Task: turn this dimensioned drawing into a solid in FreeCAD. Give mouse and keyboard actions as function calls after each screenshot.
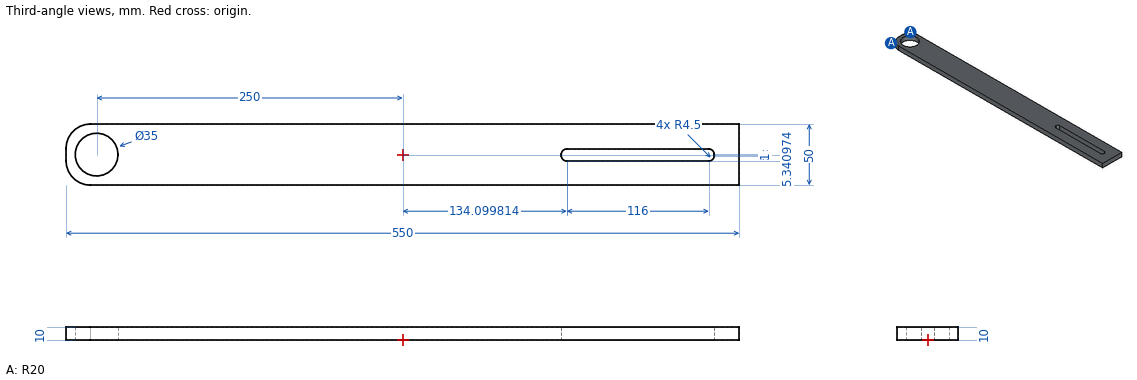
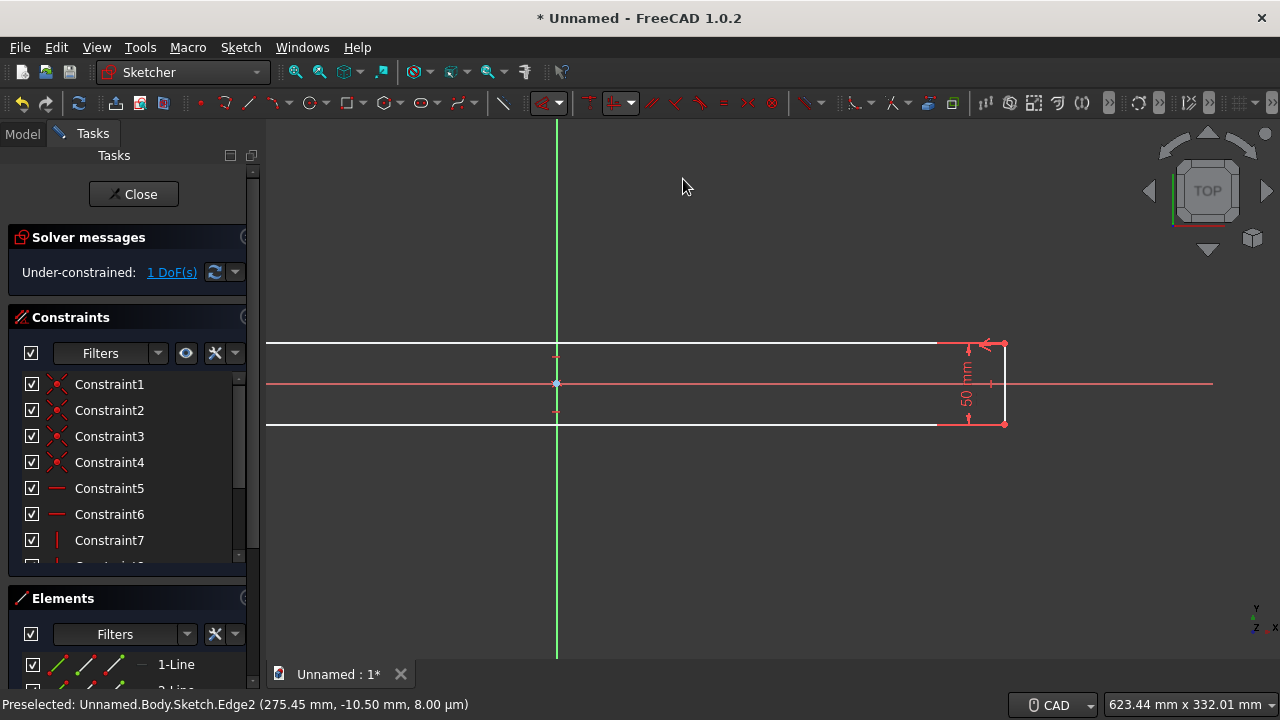
click(377, 425)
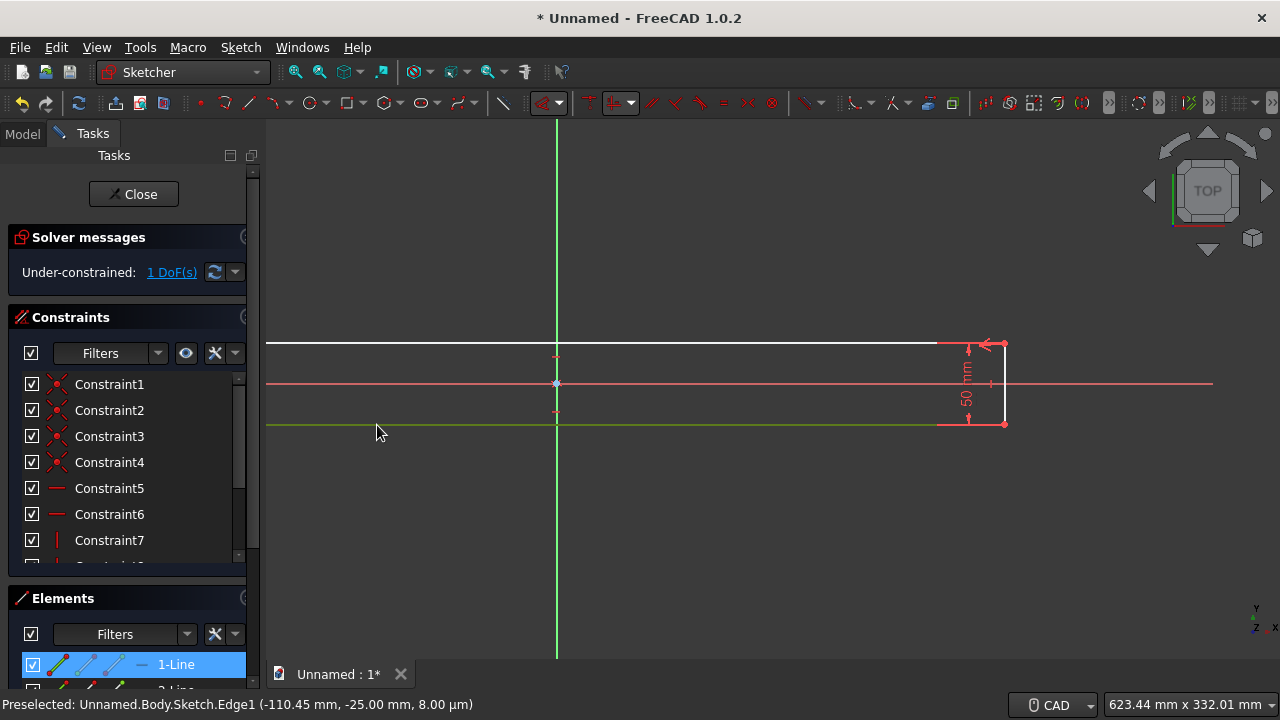
key(l)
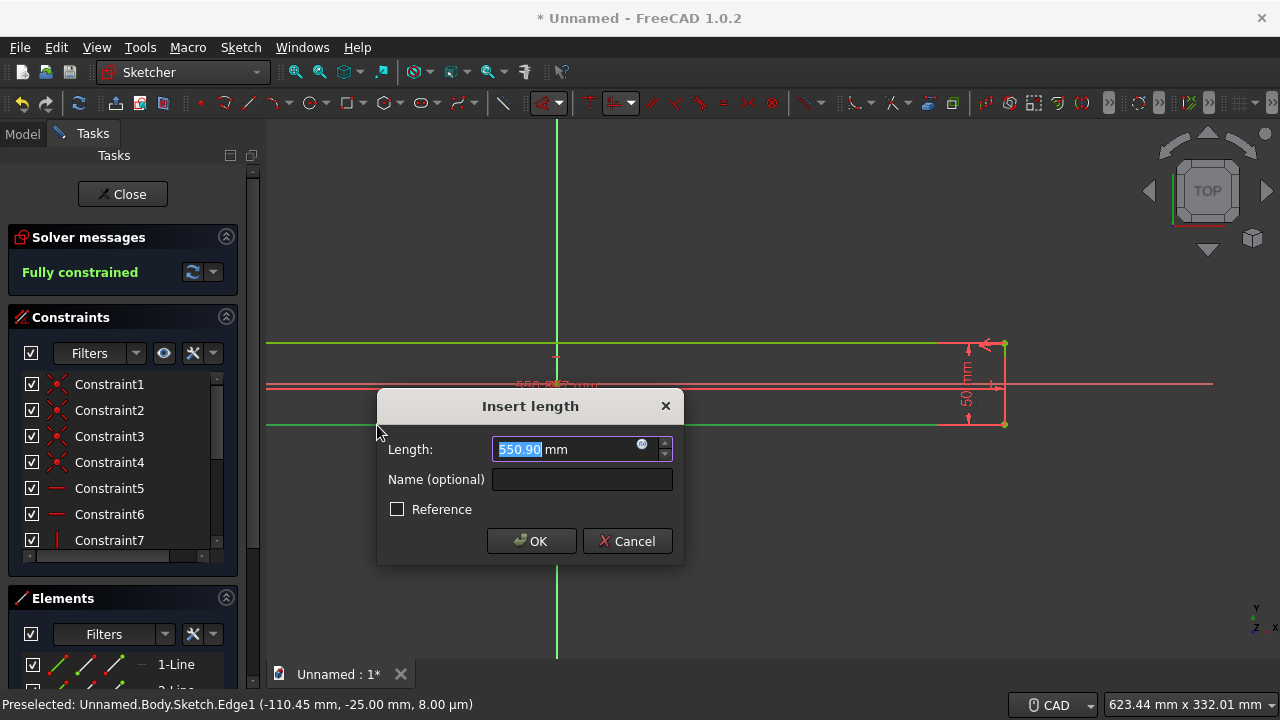
text(550)
key(Return)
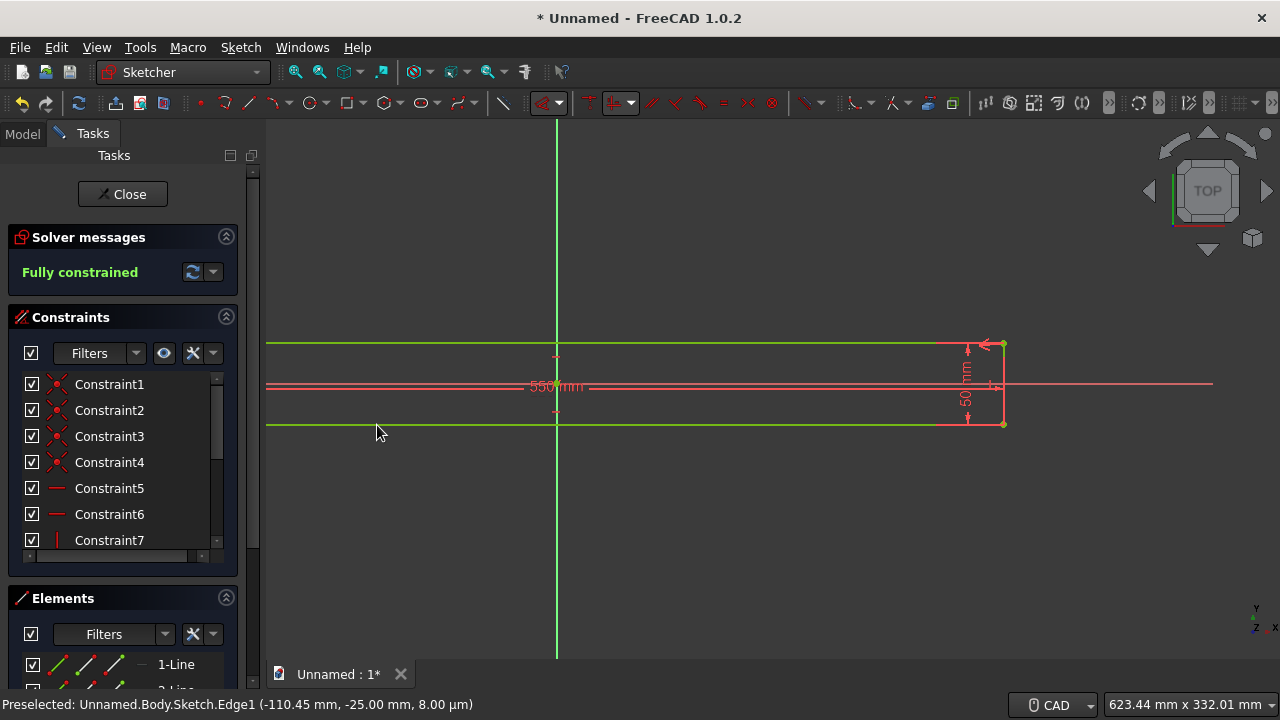
click(123, 194)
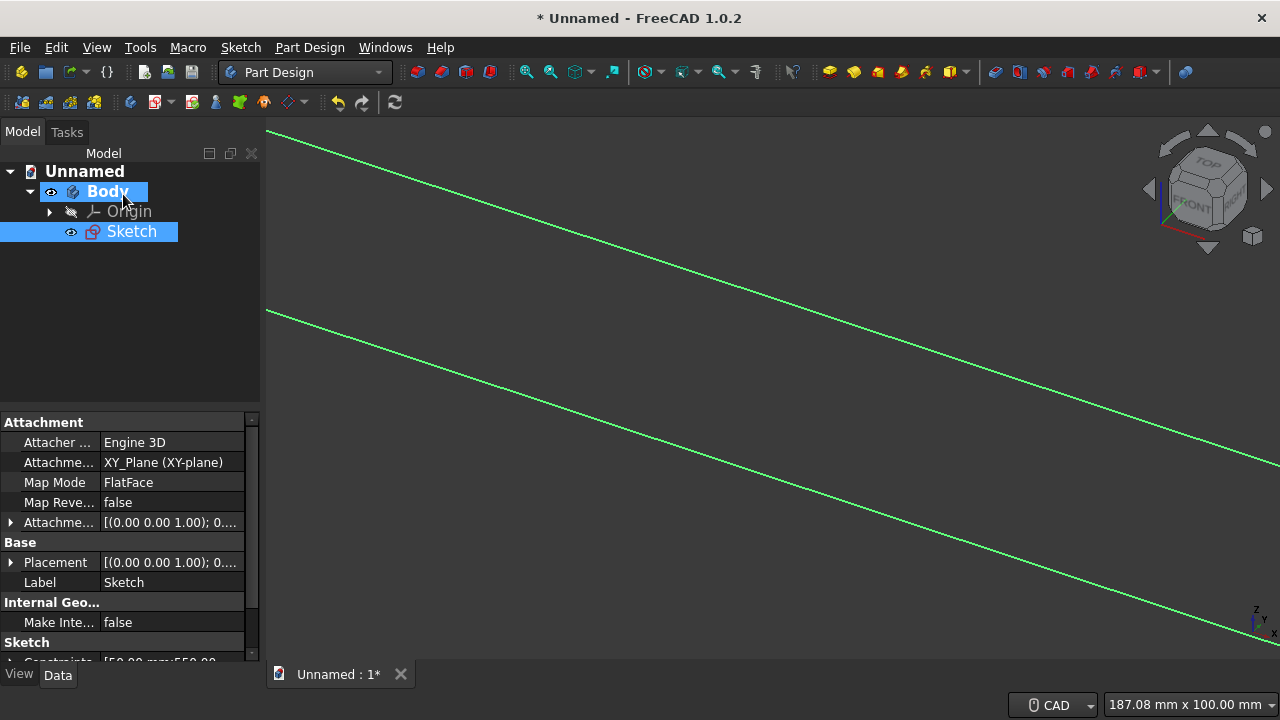
click(830, 72)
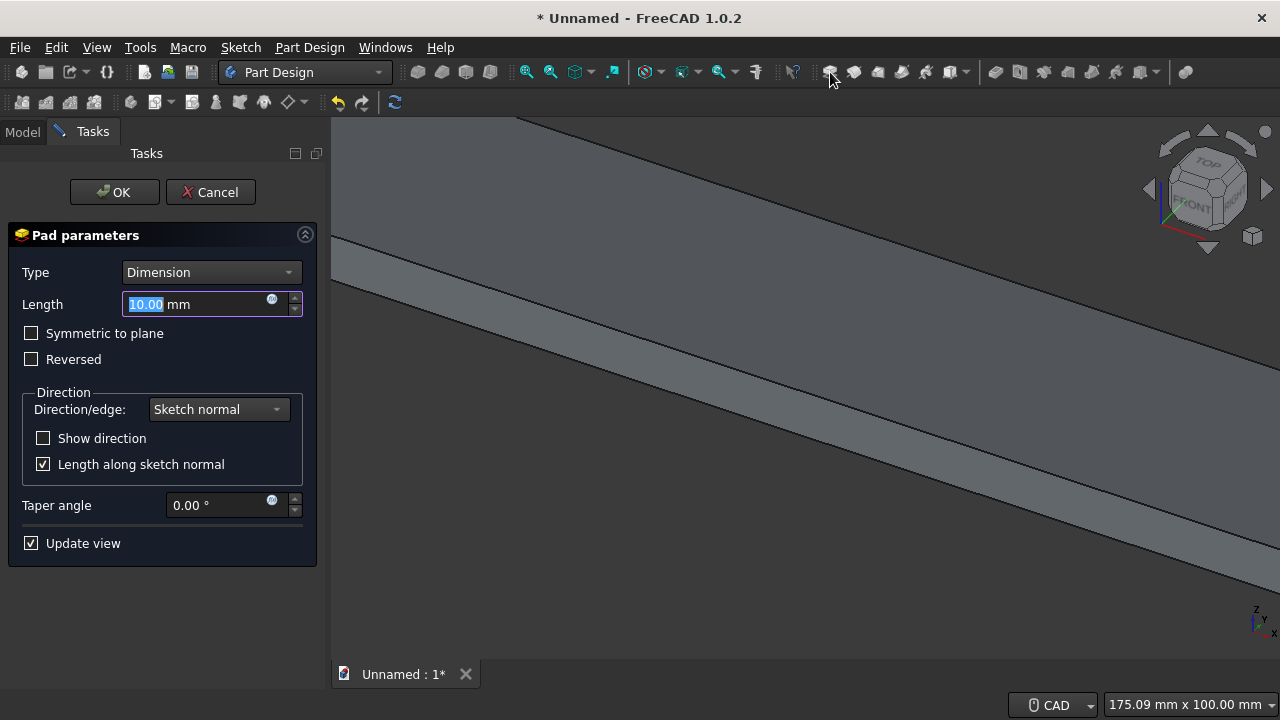
text(10)
key(Tab)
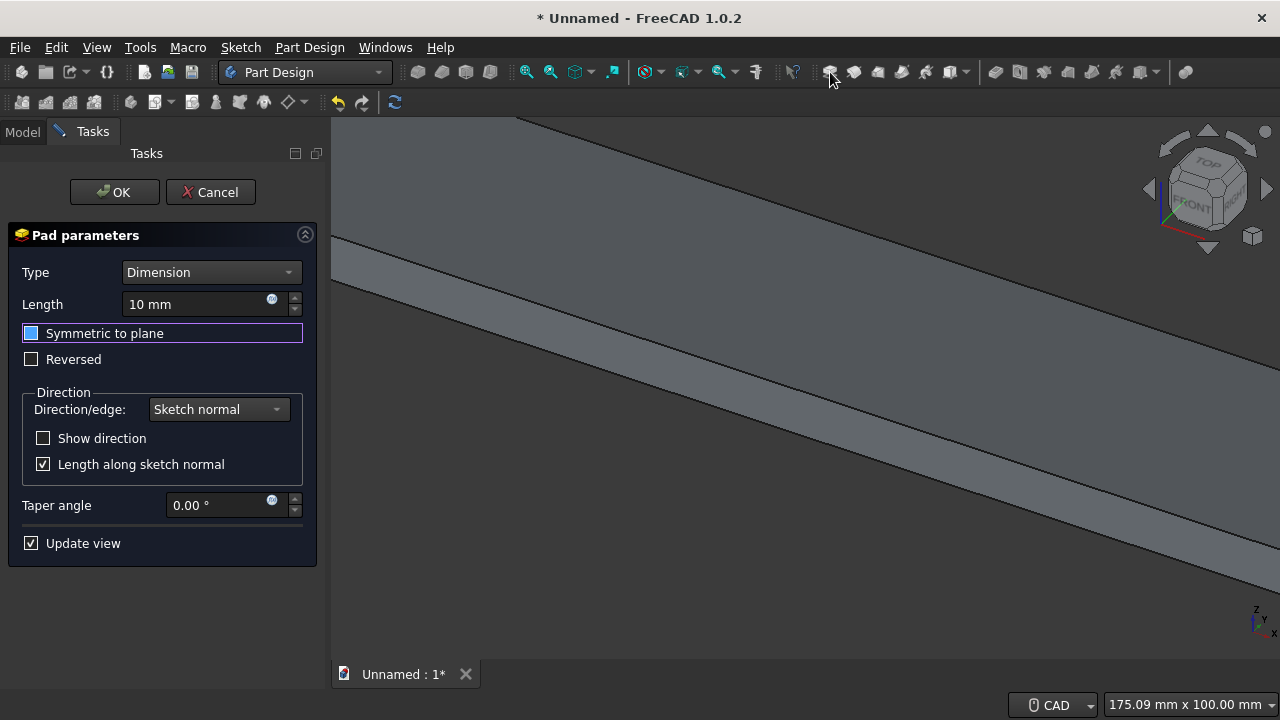
click(115, 192)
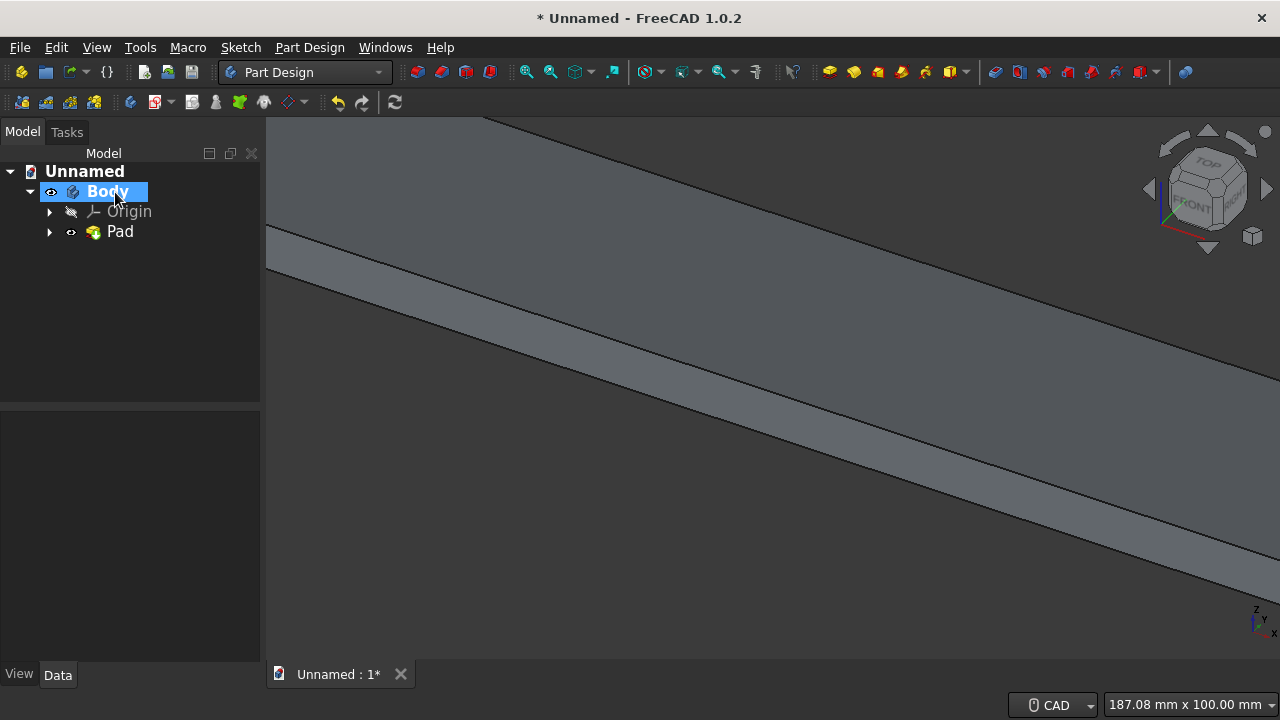
click(528, 72)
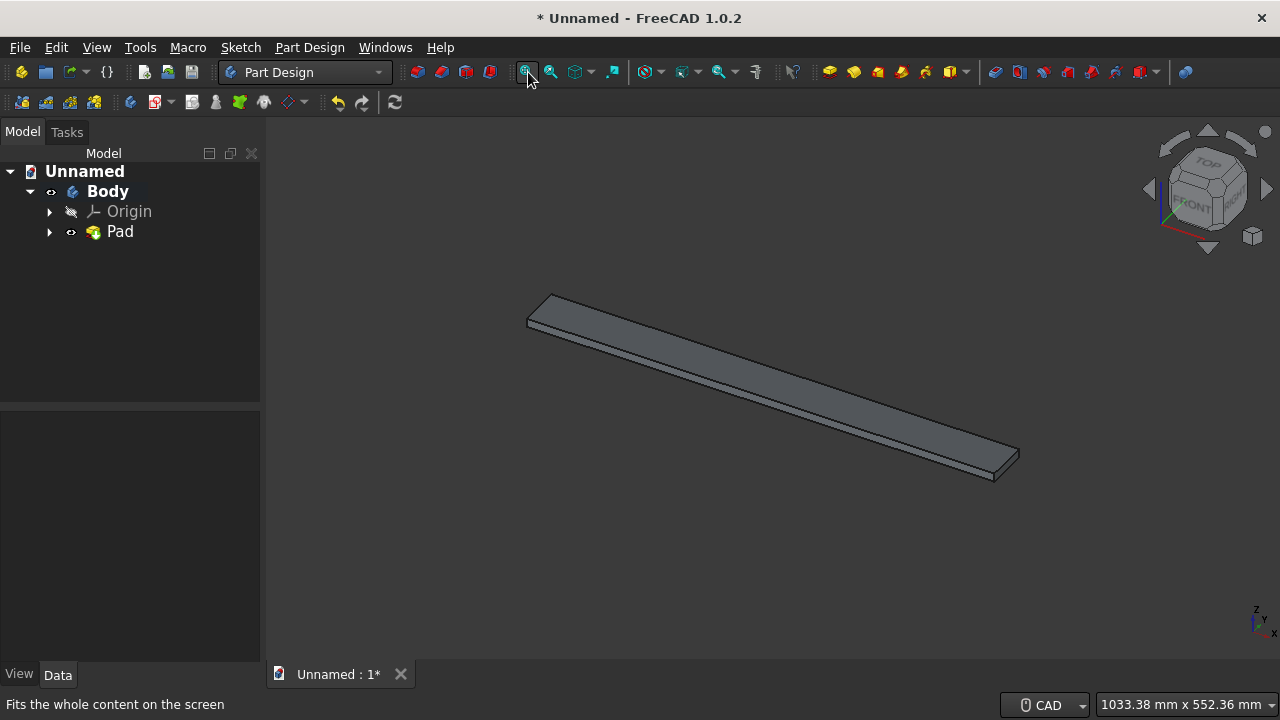
click(973, 449)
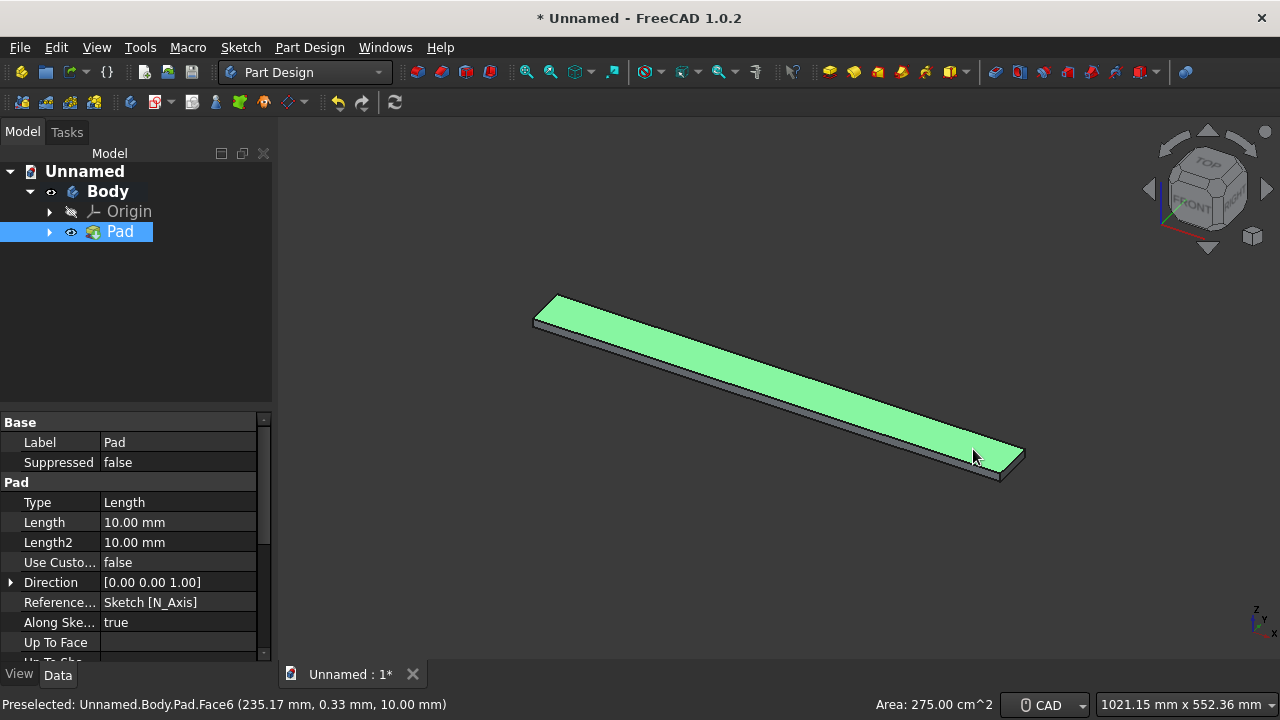
click(156, 102)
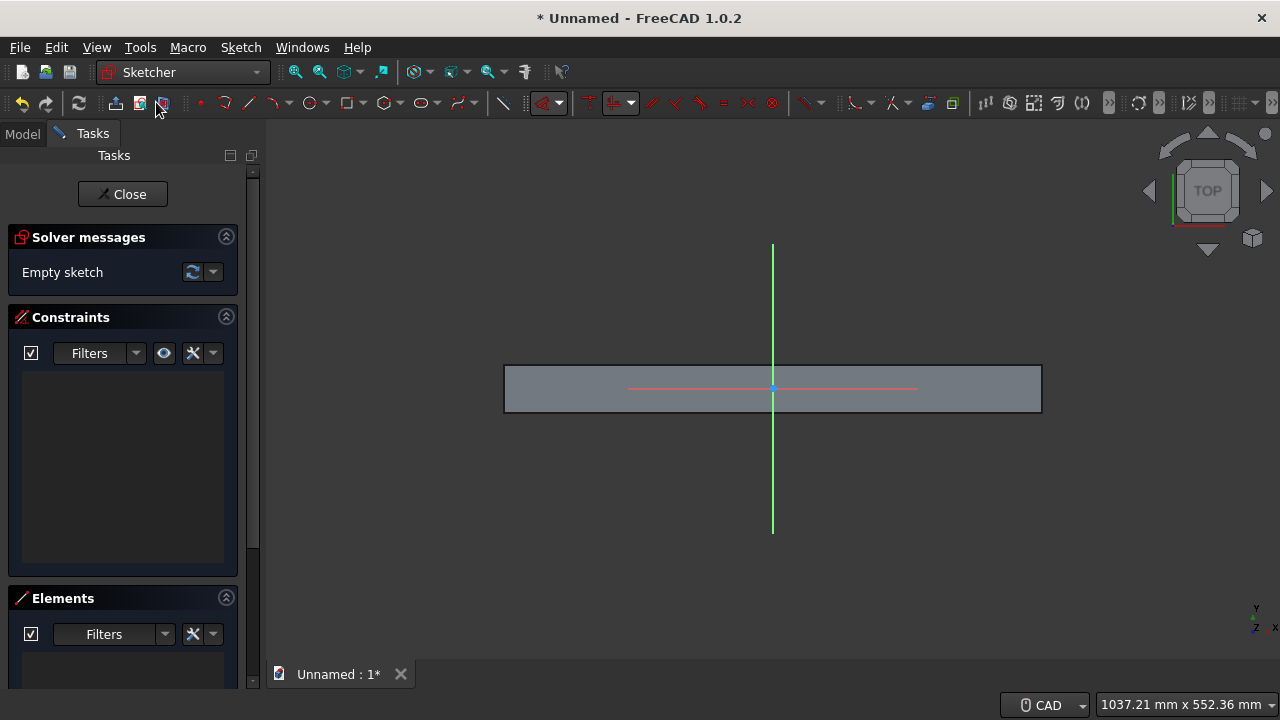
scroll(511, 389, up, 12)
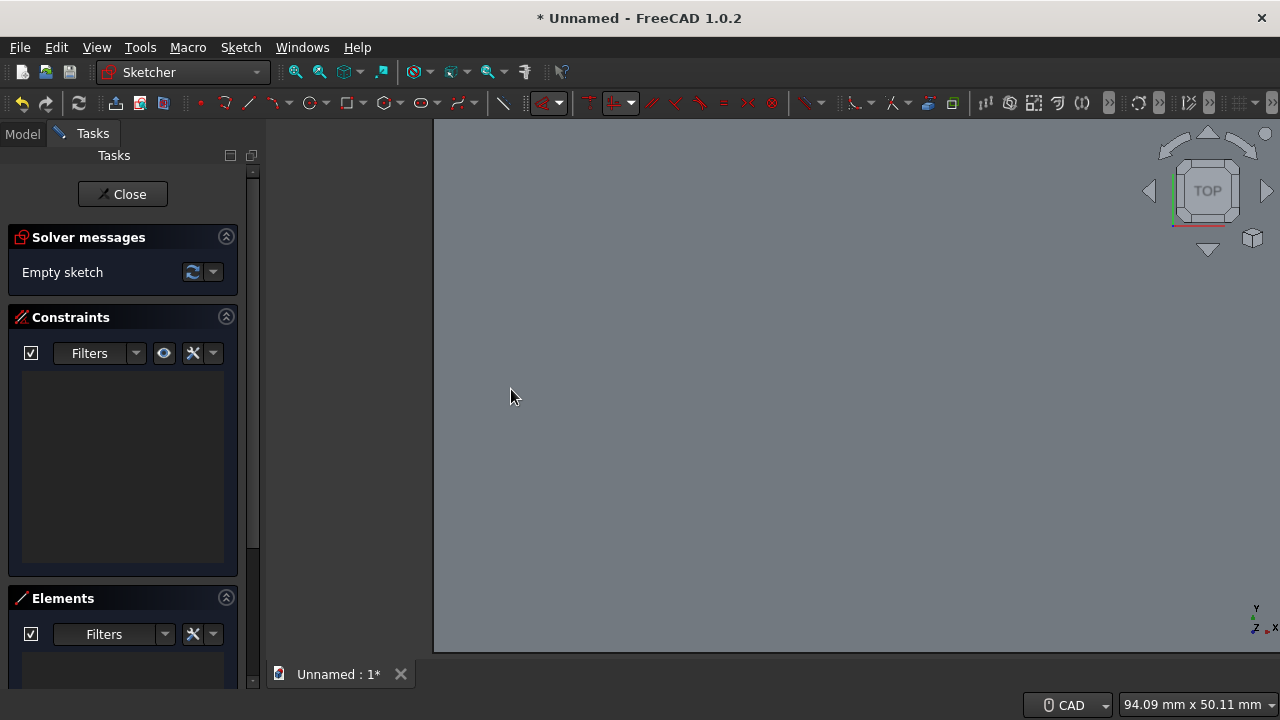
click(310, 104)